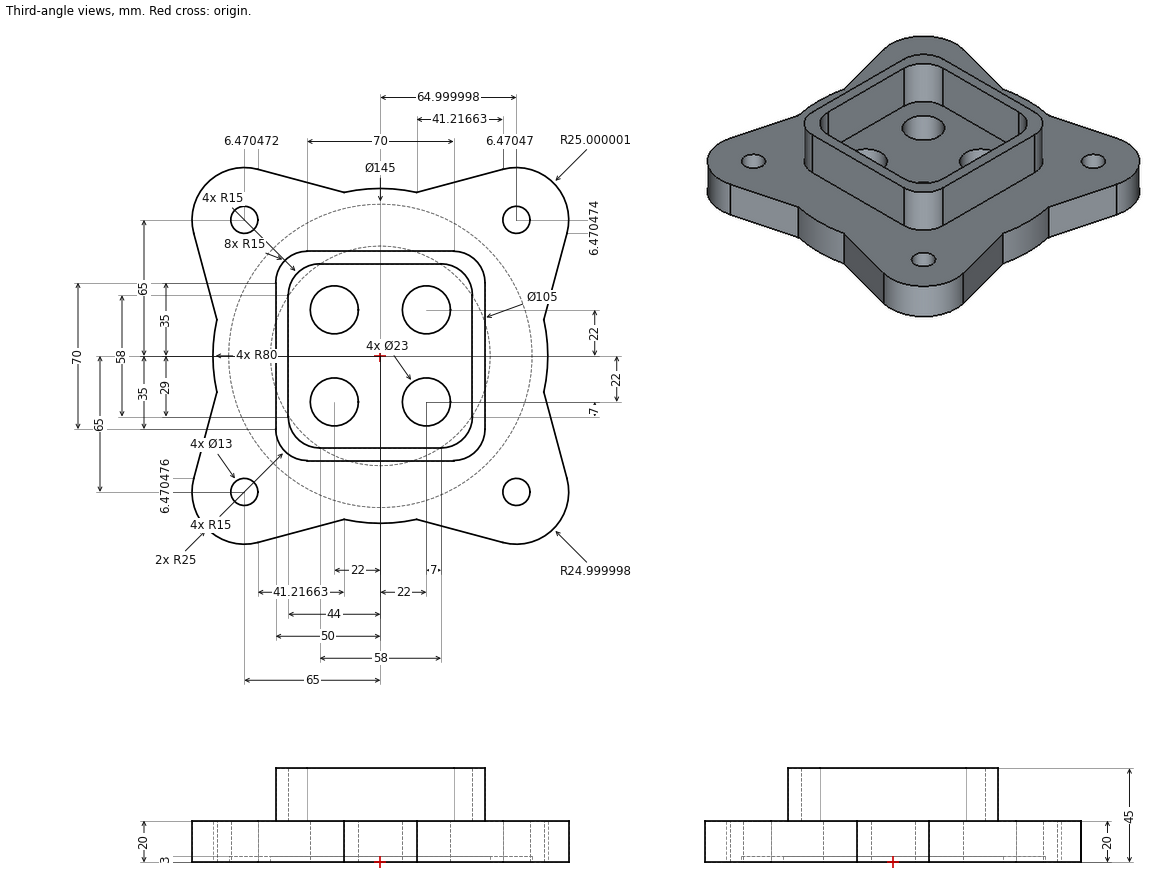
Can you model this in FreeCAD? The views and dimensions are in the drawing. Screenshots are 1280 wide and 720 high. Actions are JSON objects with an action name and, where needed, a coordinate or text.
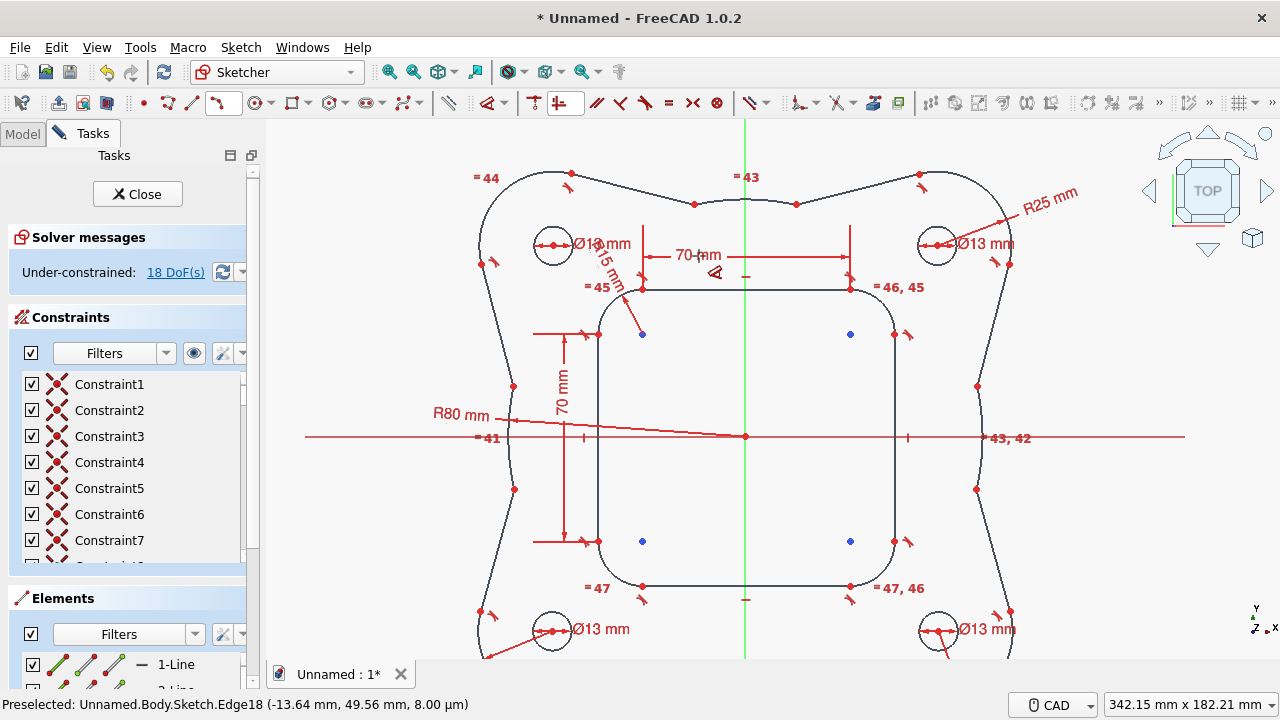
{"action": "scroll", "coordinate": [621, 292], "scroll_direction": "down", "scroll_amount": 2}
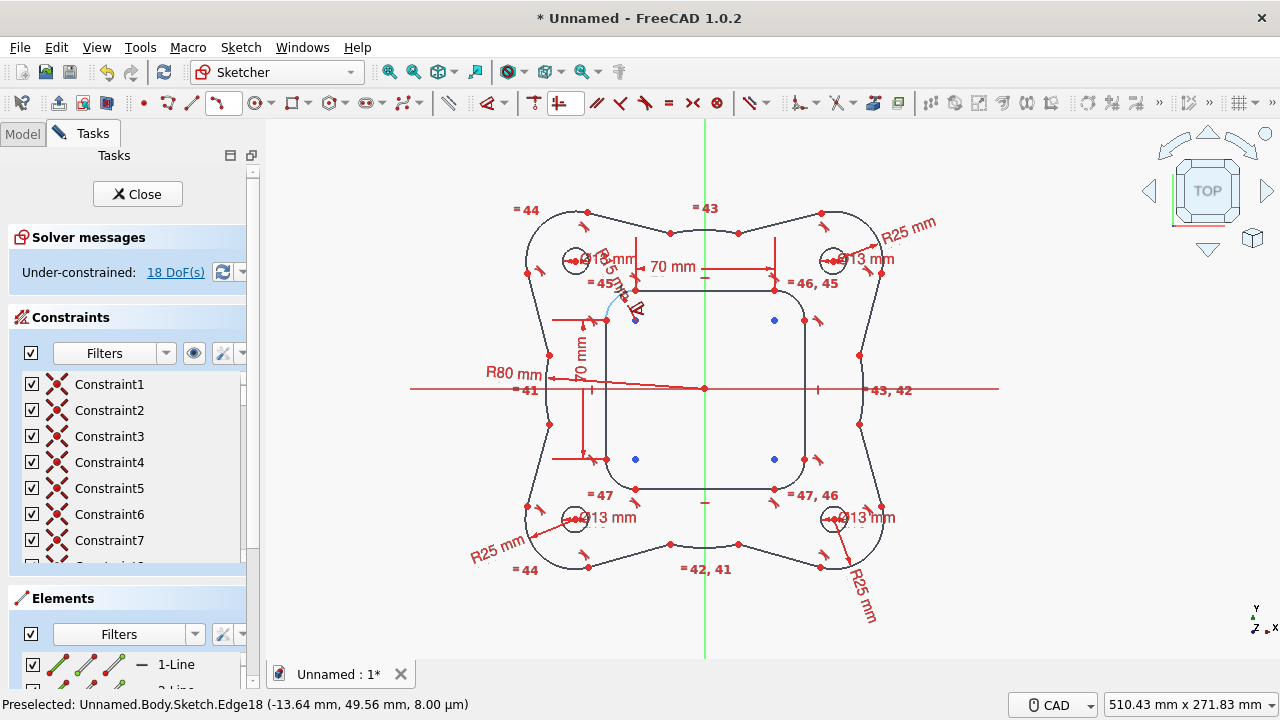
{"action": "left_click", "coordinate": [575, 520]}
{"action": "left_click", "coordinate": [670, 355]}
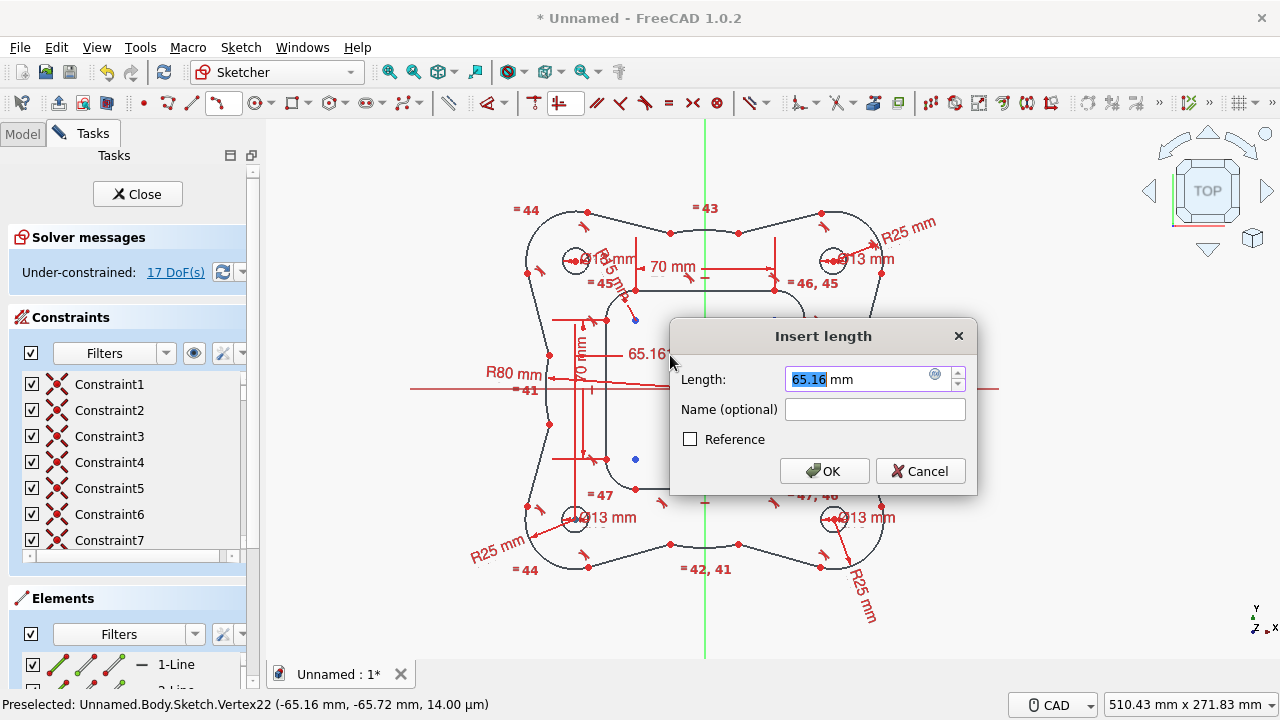
{"action": "type", "text": "65"}
{"action": "key", "text": "Return"}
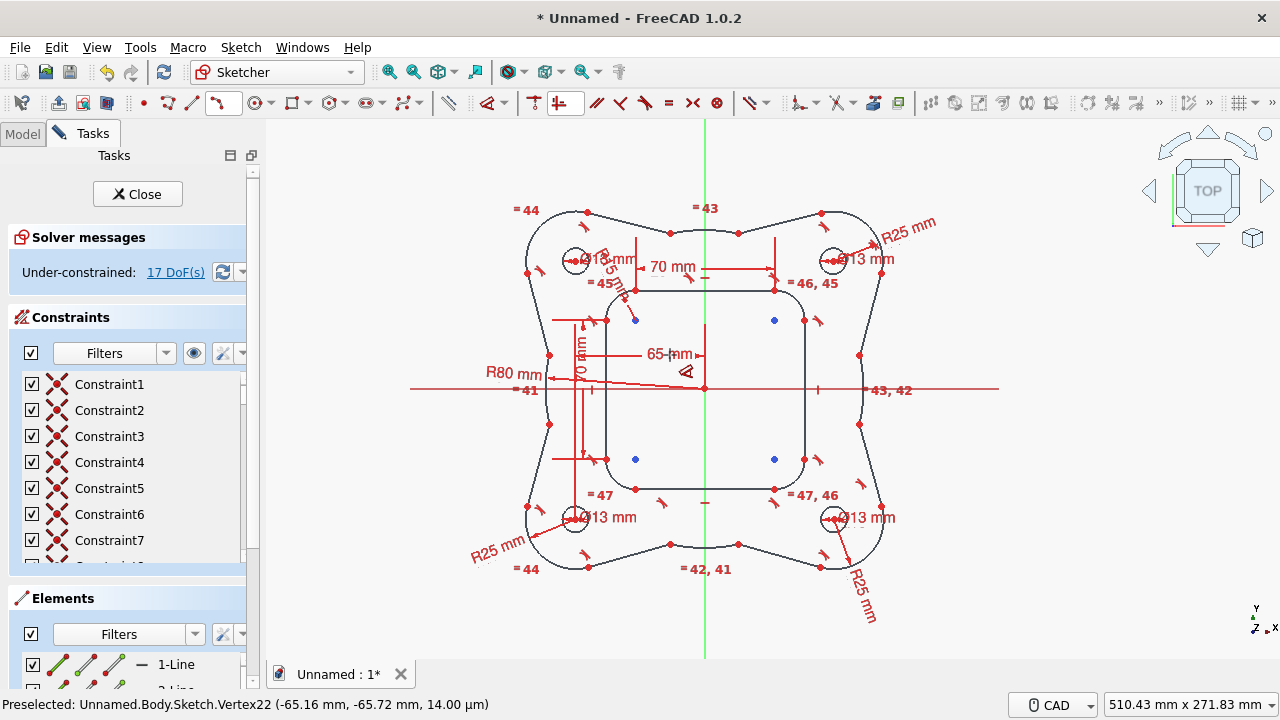
{"action": "left_click", "coordinate": [575, 519]}
{"action": "left_click", "coordinate": [739, 454]}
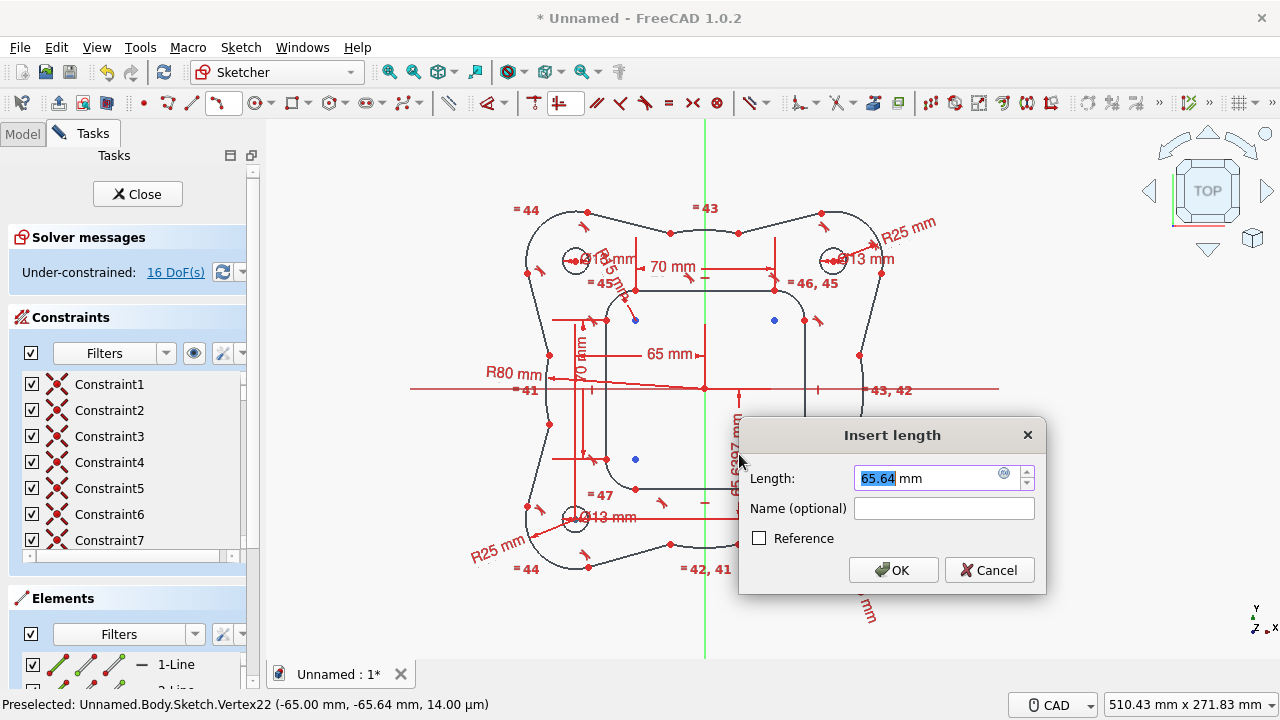
{"action": "type", "text": "65"}
{"action": "key", "text": "Return"}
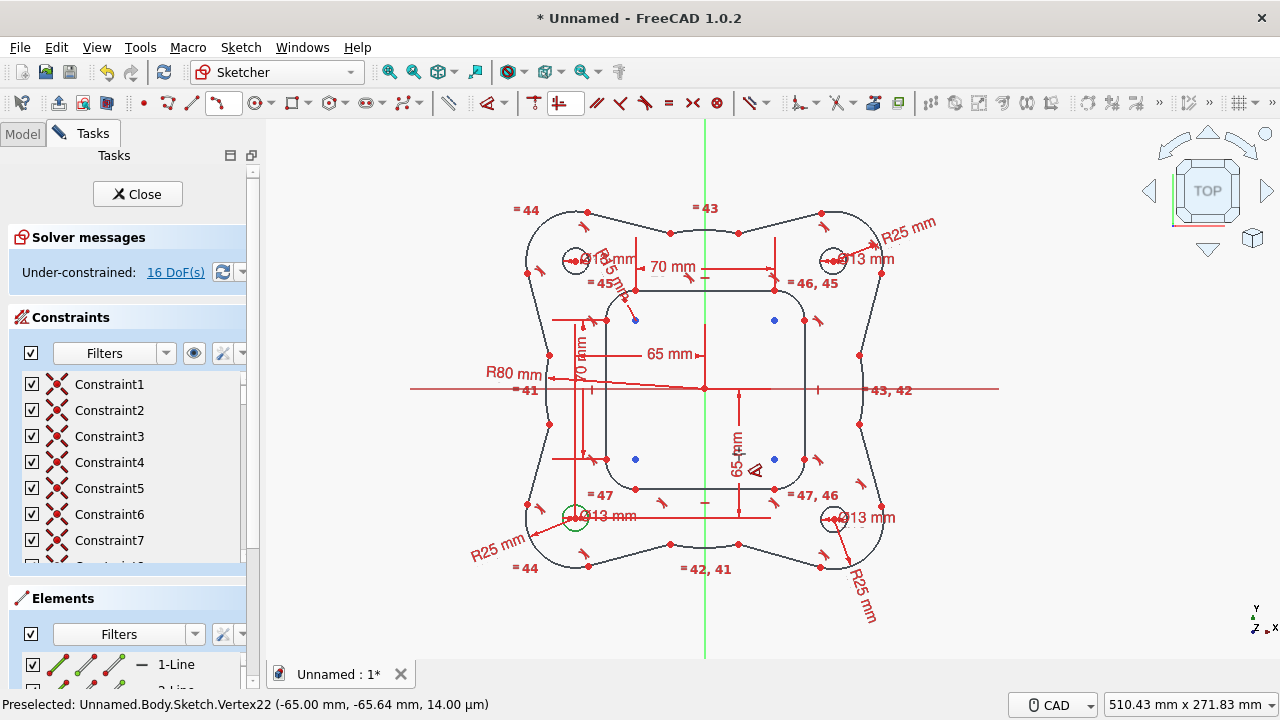
{"action": "left_click", "coordinate": [576, 261]}
{"action": "left_click", "coordinate": [640, 423]}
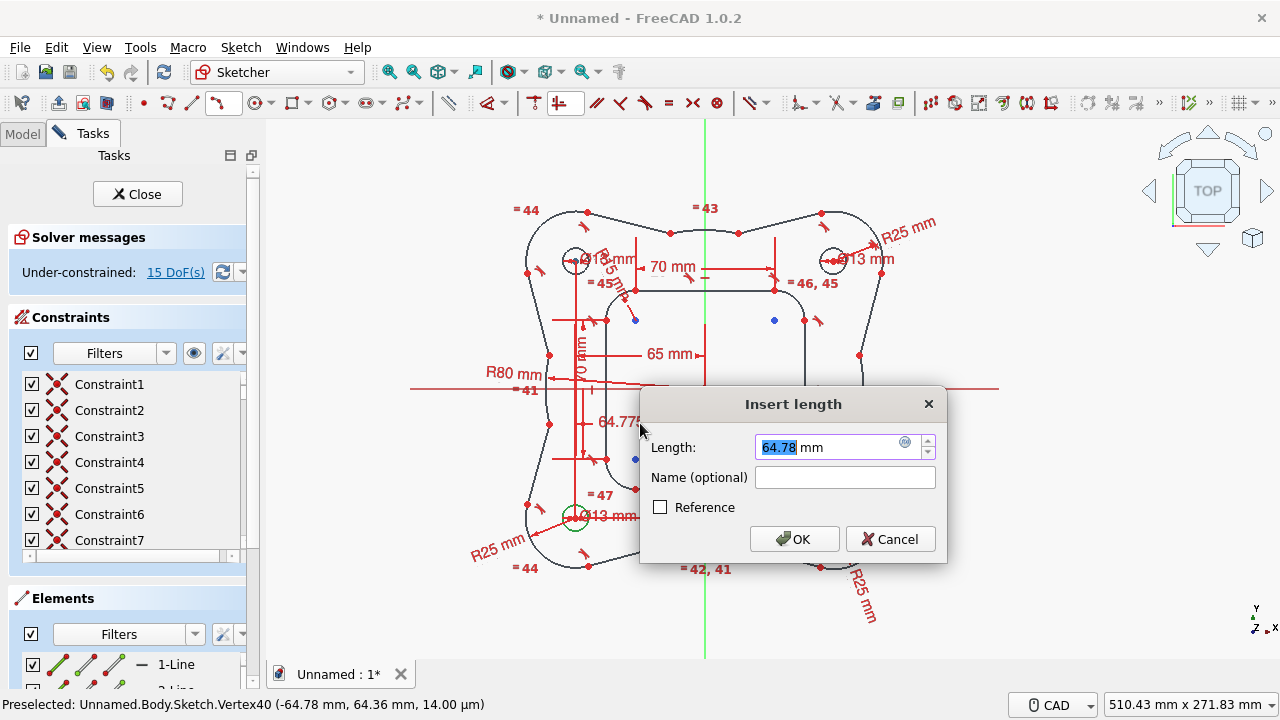
{"action": "type", "text": "65"}
{"action": "key", "text": "Return"}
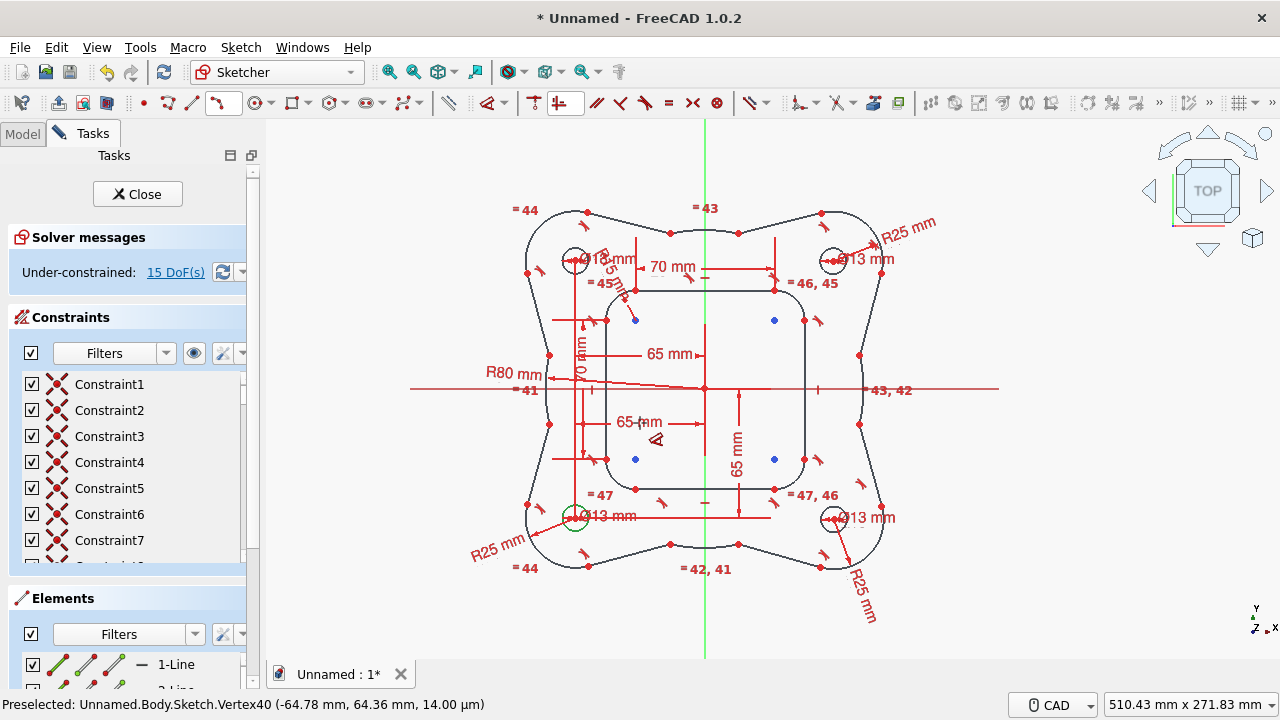
{"action": "left_click", "coordinate": [575, 261]}
{"action": "left_click", "coordinate": [739, 325]}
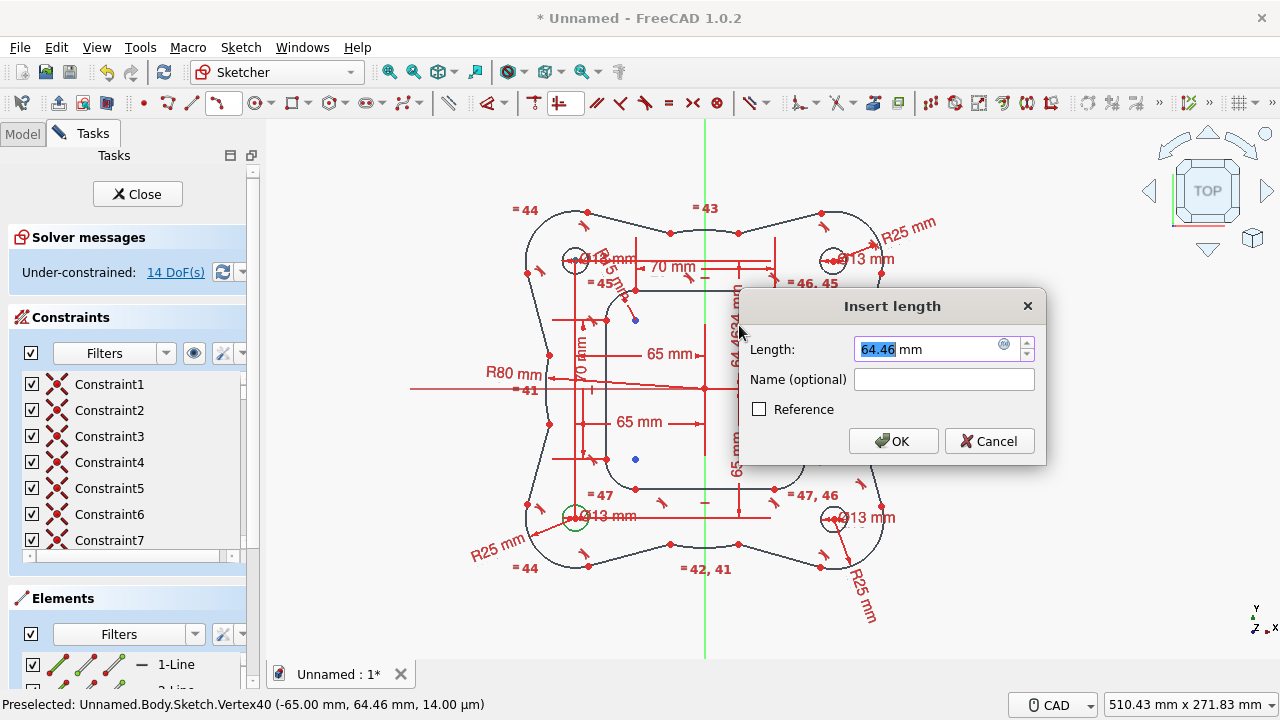
{"action": "type", "text": "65"}
{"action": "key", "text": "Return"}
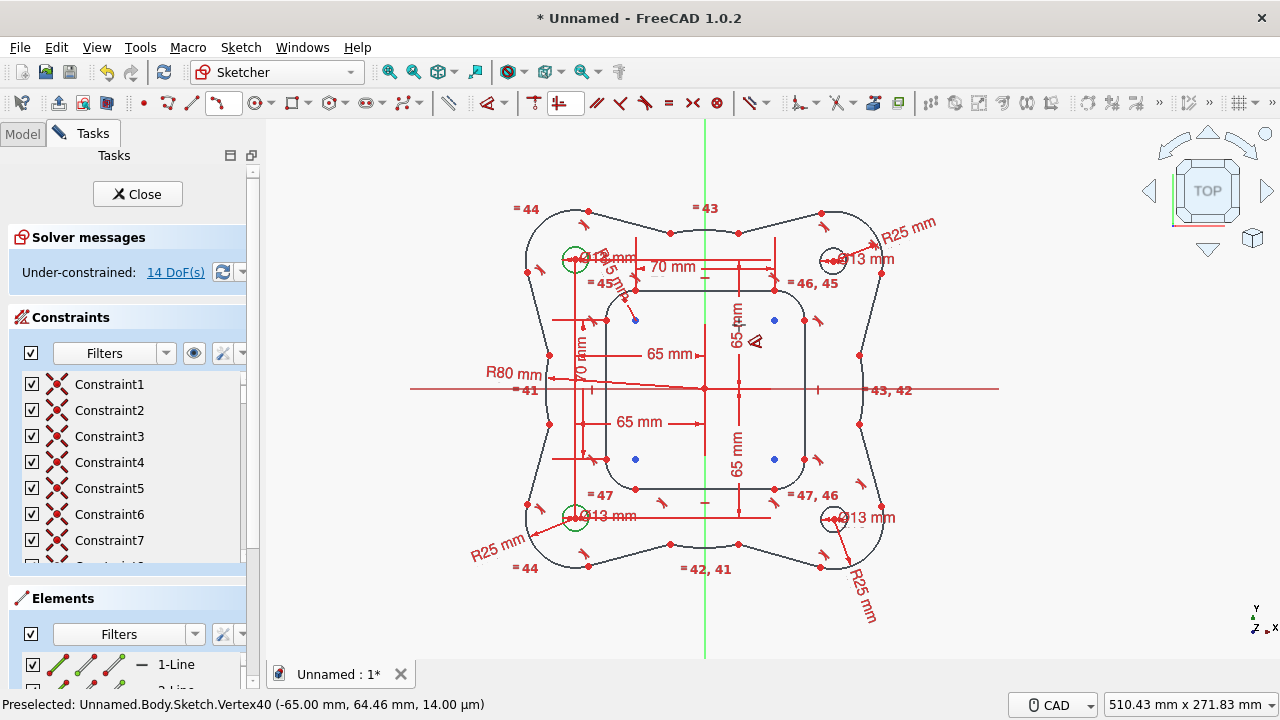
{"action": "left_click", "coordinate": [606, 459]}
{"action": "left_click", "coordinate": [655, 517]}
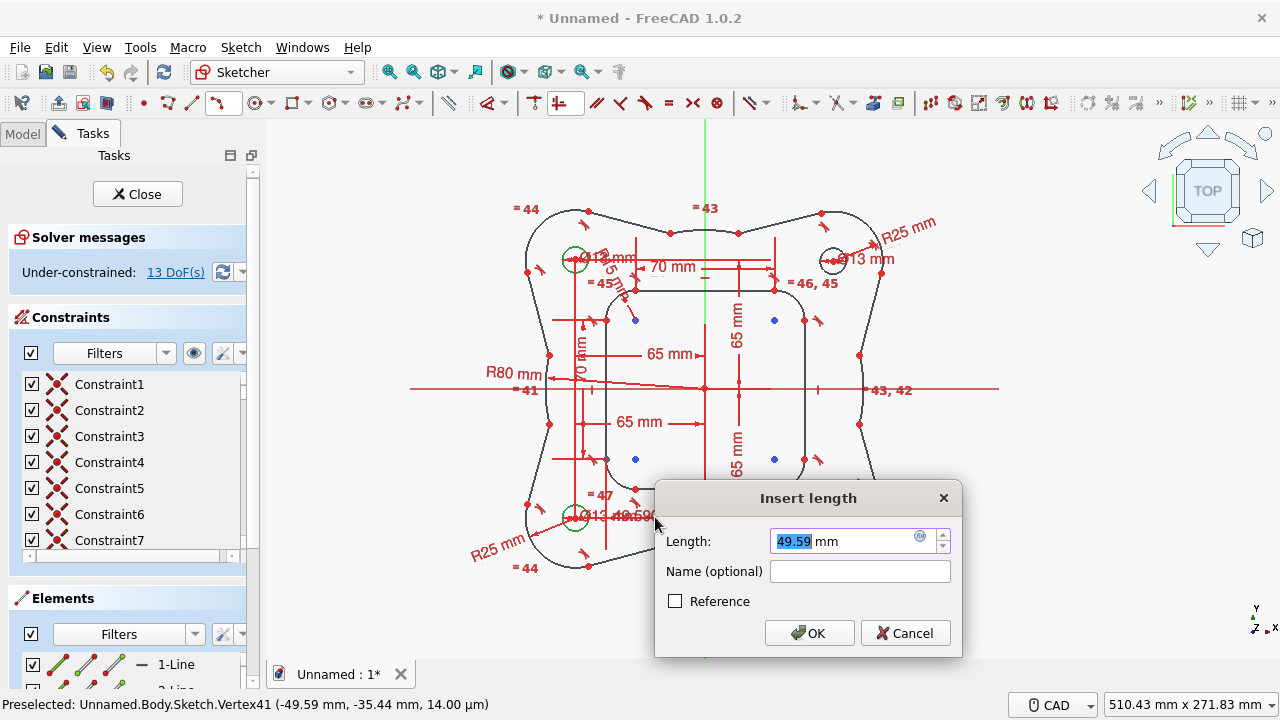
{"action": "type", "text": "50"}
{"action": "key", "text": "Return"}